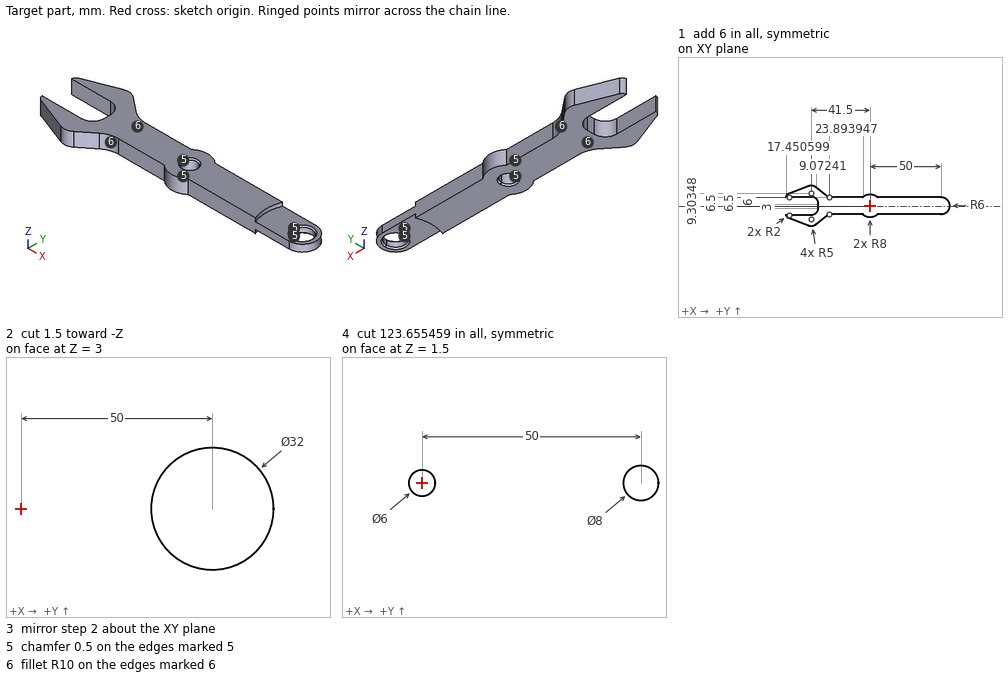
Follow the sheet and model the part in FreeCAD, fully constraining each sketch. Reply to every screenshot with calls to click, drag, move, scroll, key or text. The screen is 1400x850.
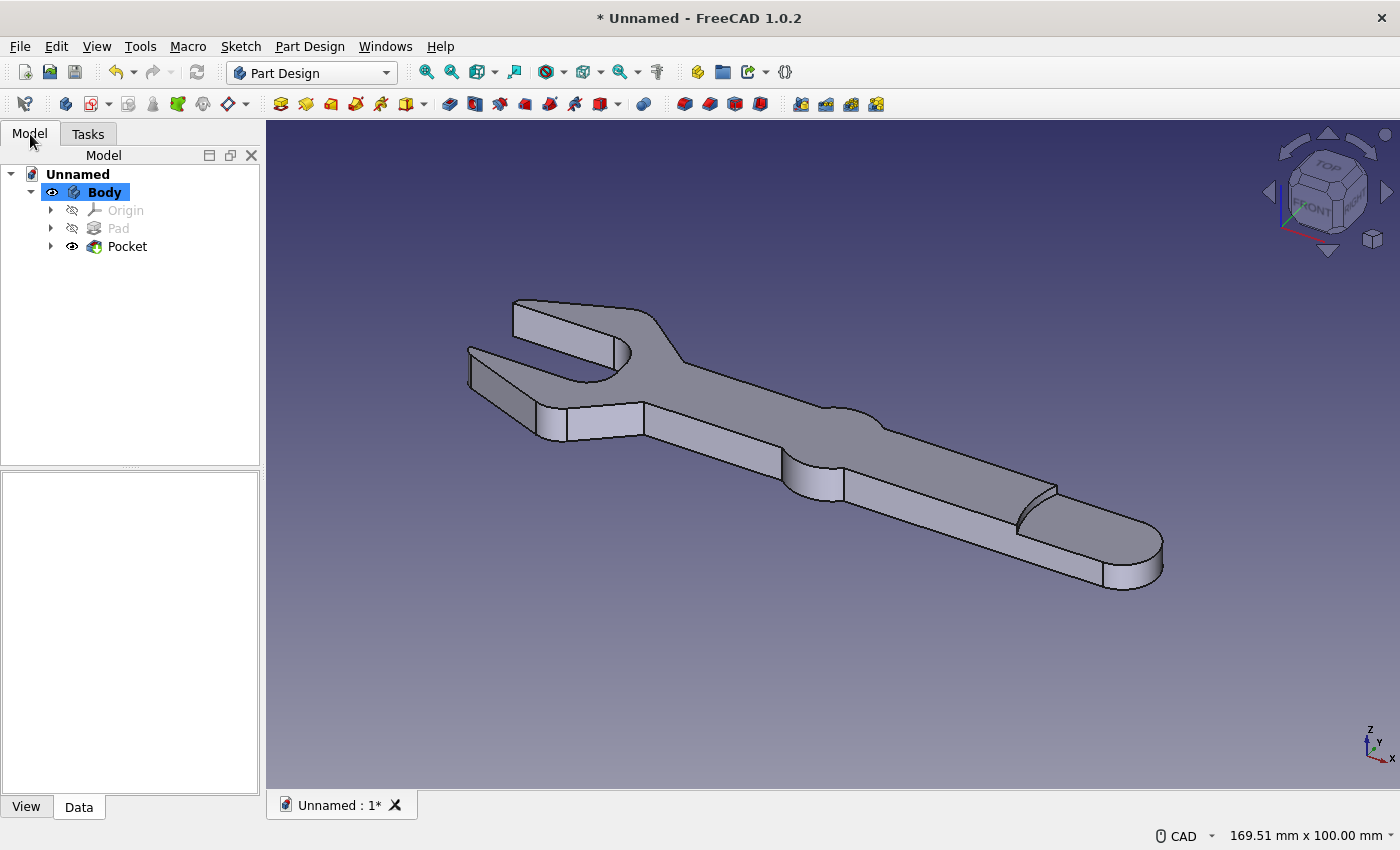
click(117, 246)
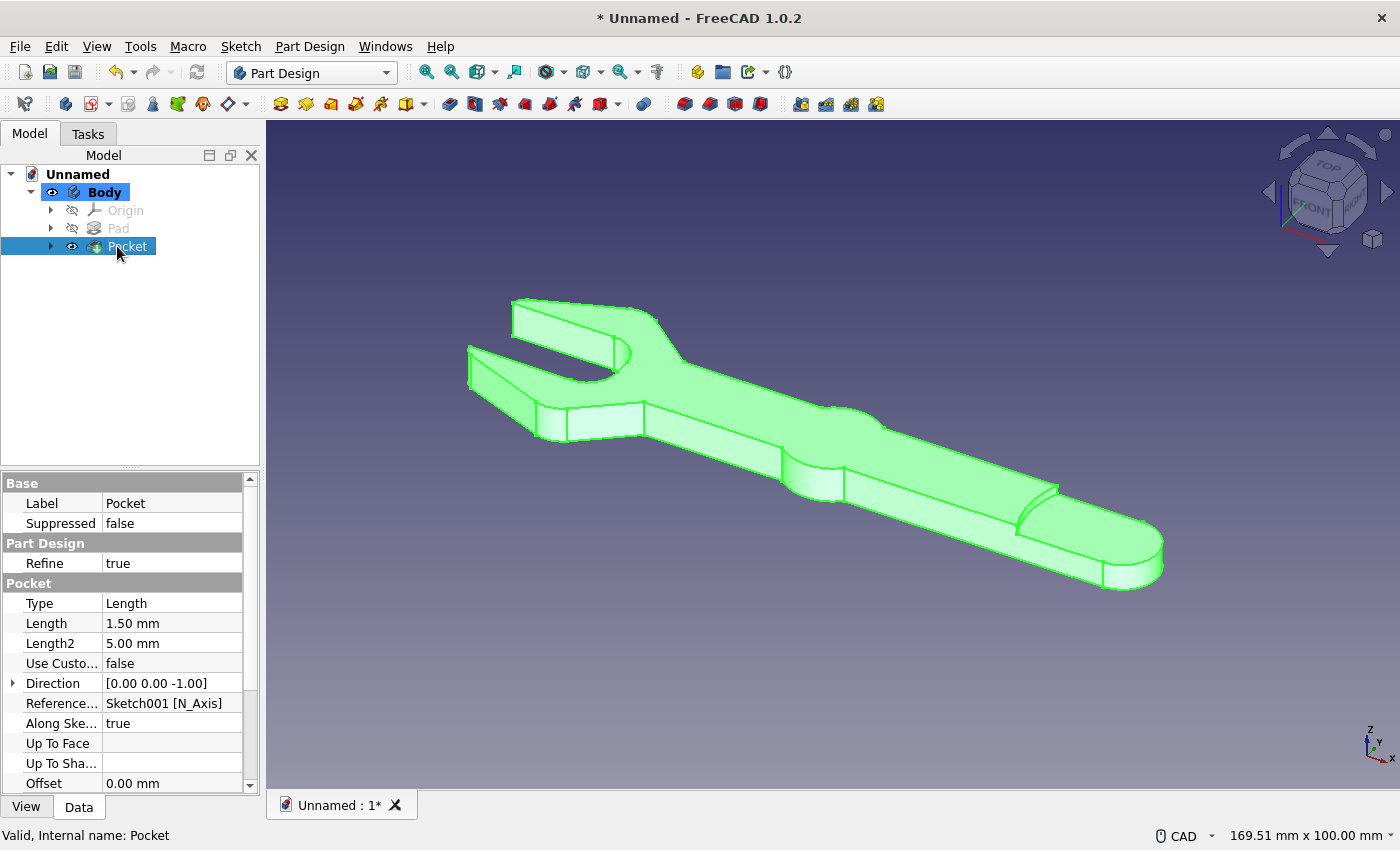
click(801, 104)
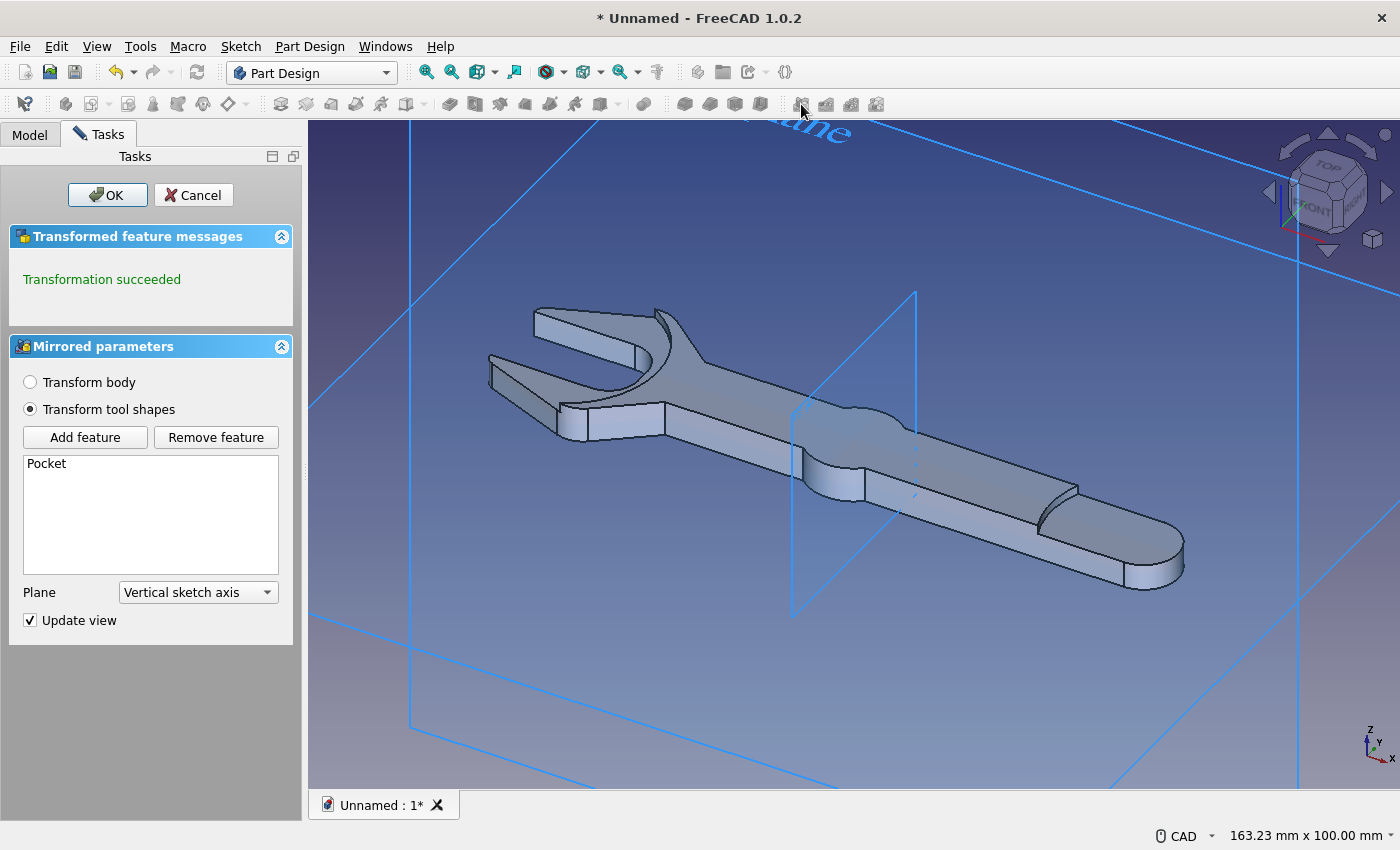
click(199, 592)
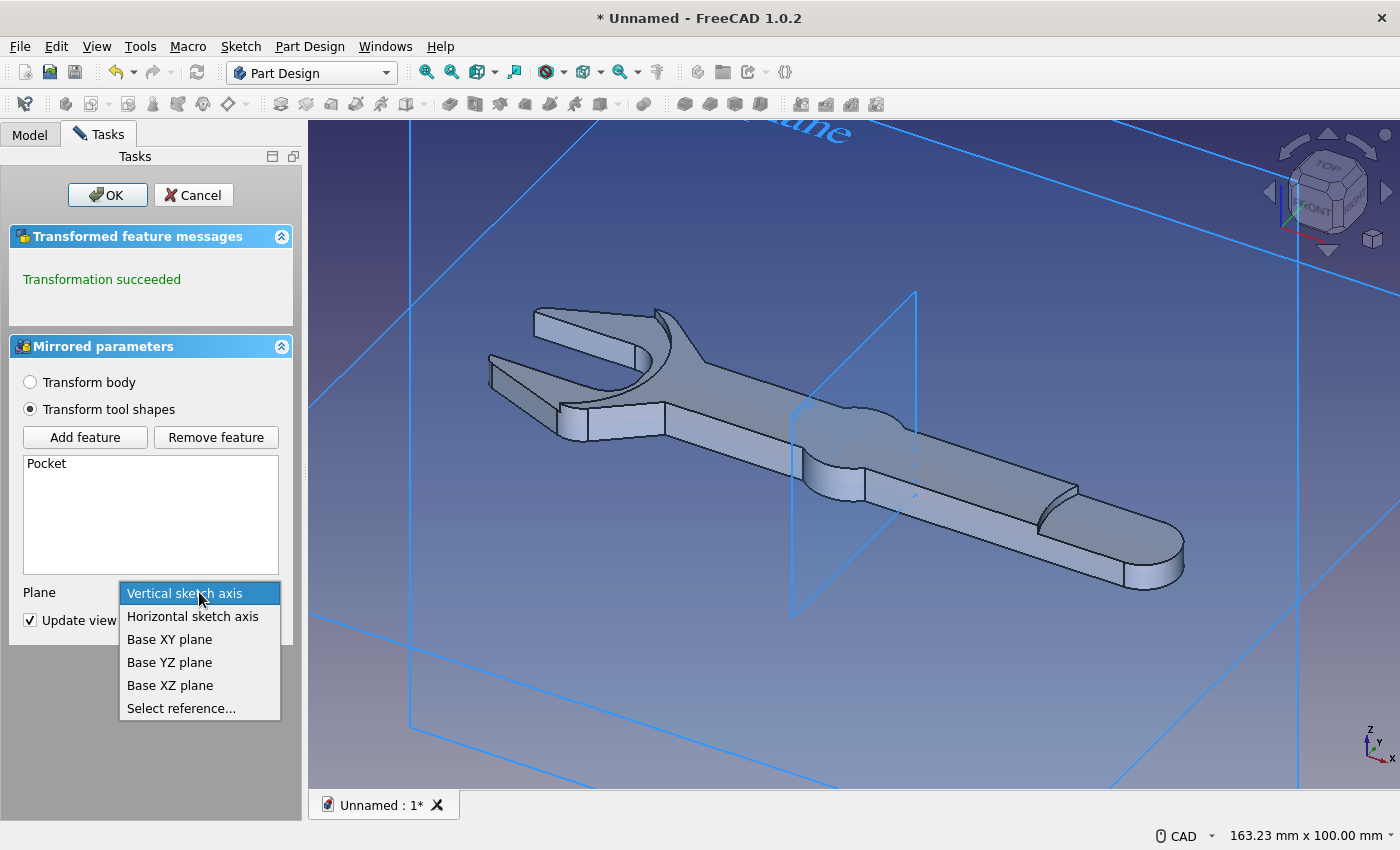
click(198, 640)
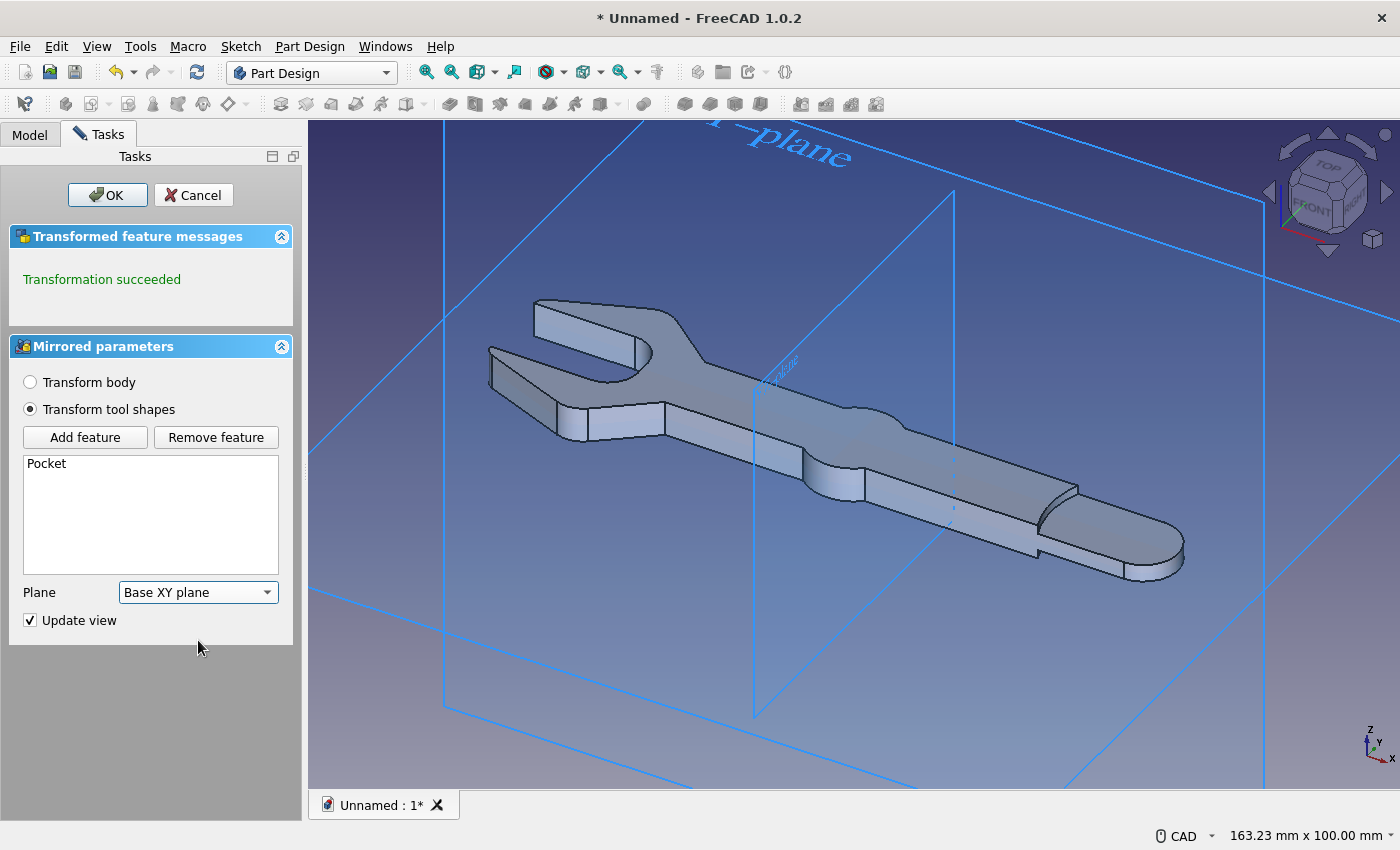
click(108, 195)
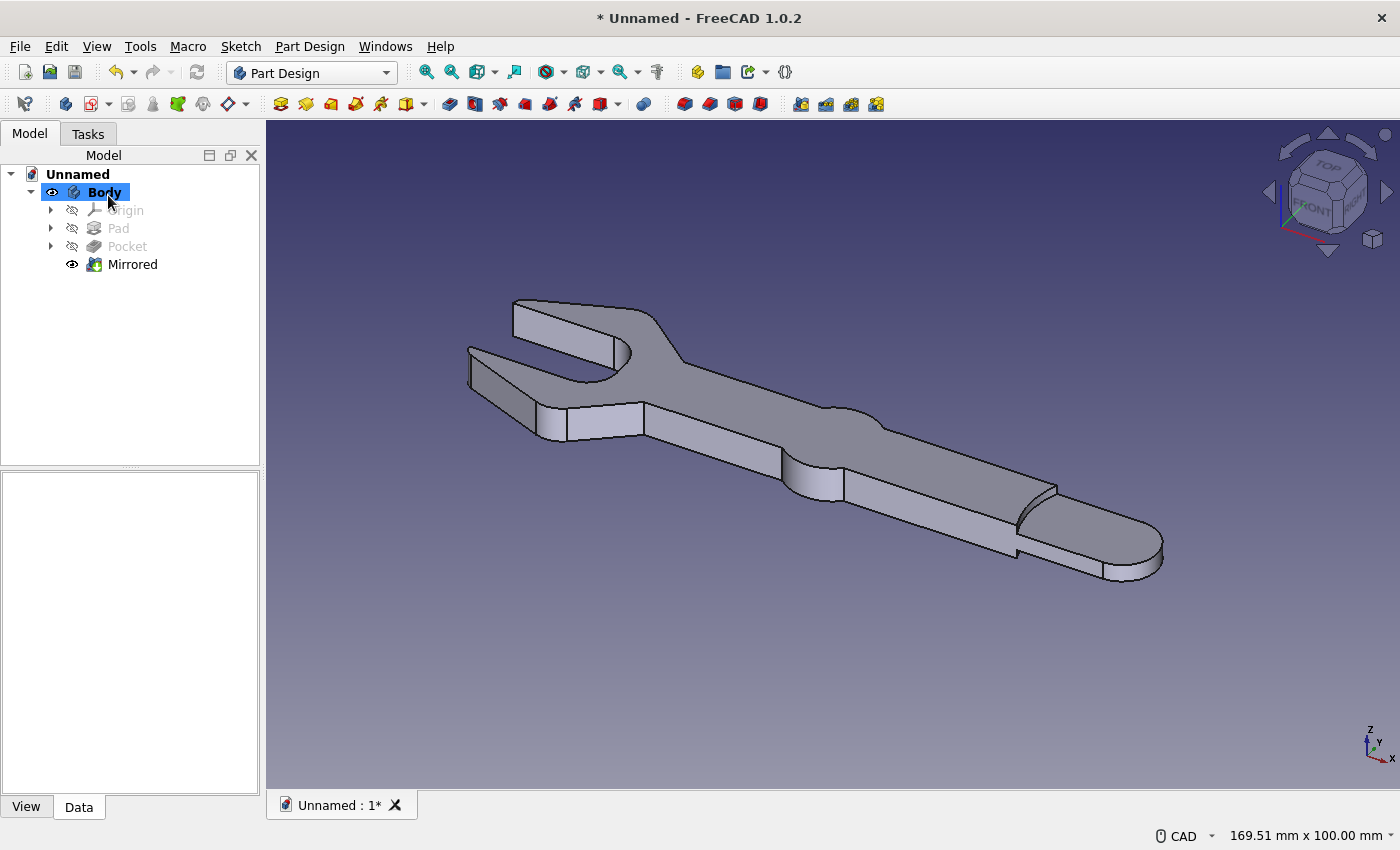
click(1112, 538)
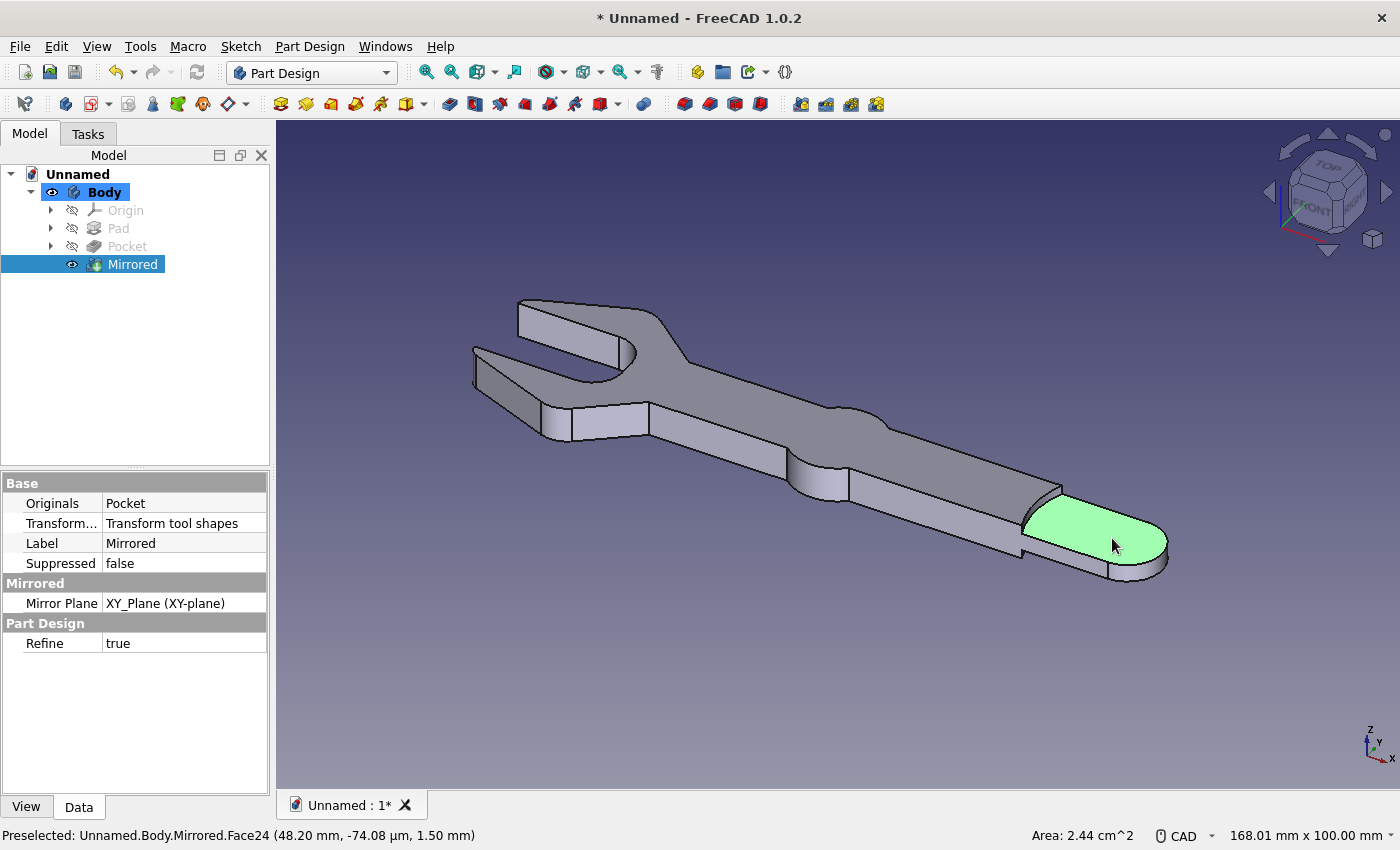
click(90, 104)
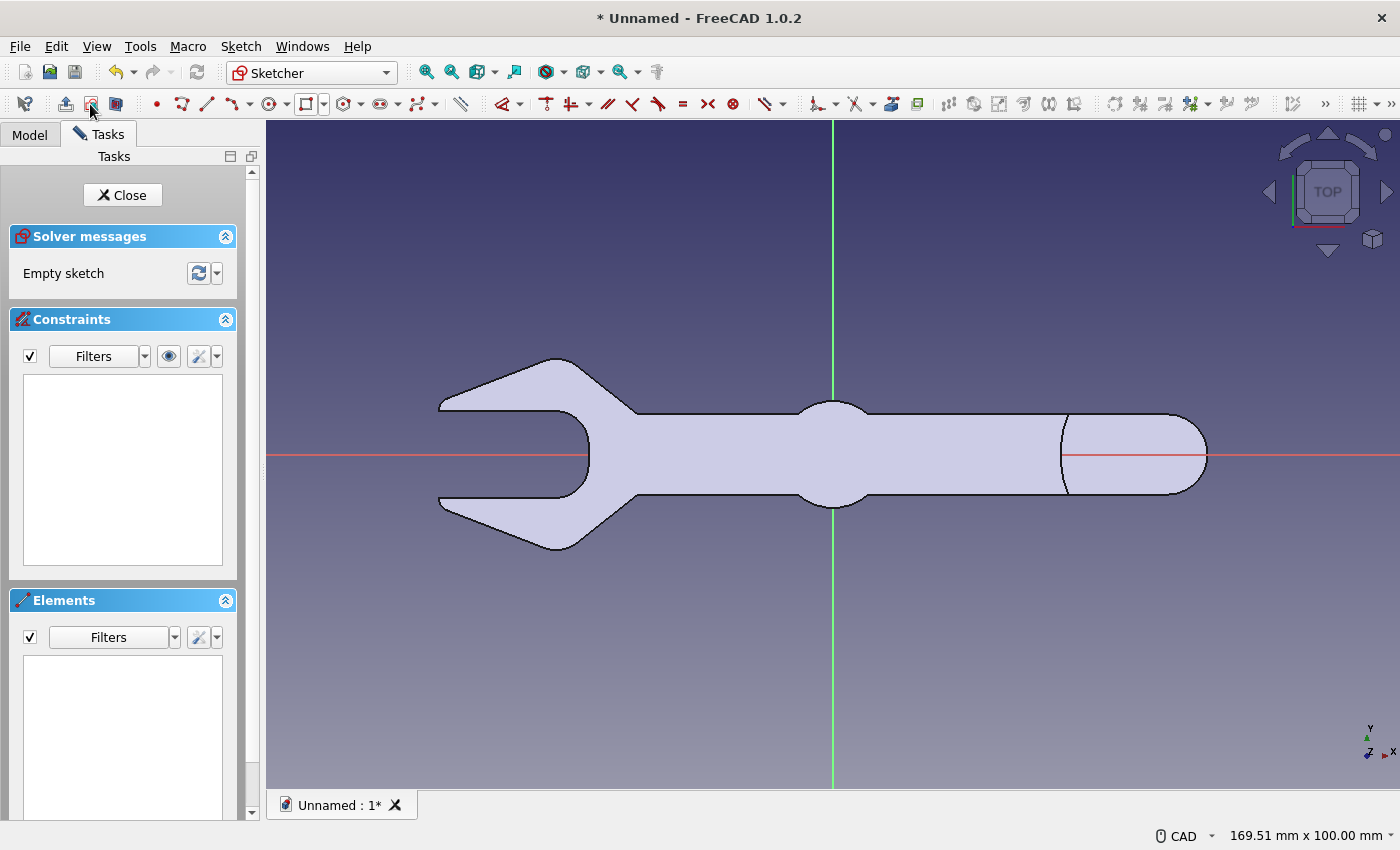
scroll(1235, 454, up, 3)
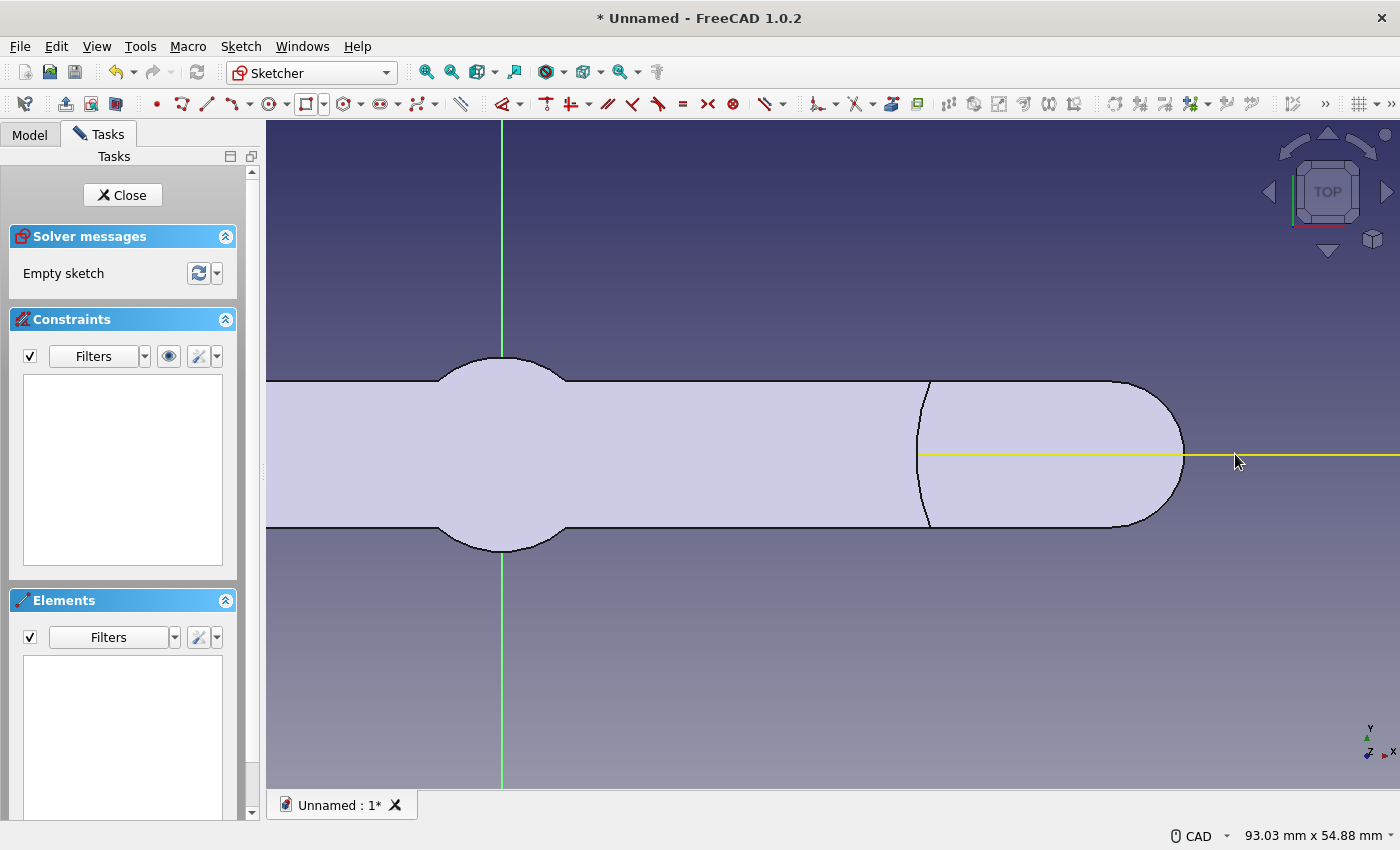
click(268, 104)